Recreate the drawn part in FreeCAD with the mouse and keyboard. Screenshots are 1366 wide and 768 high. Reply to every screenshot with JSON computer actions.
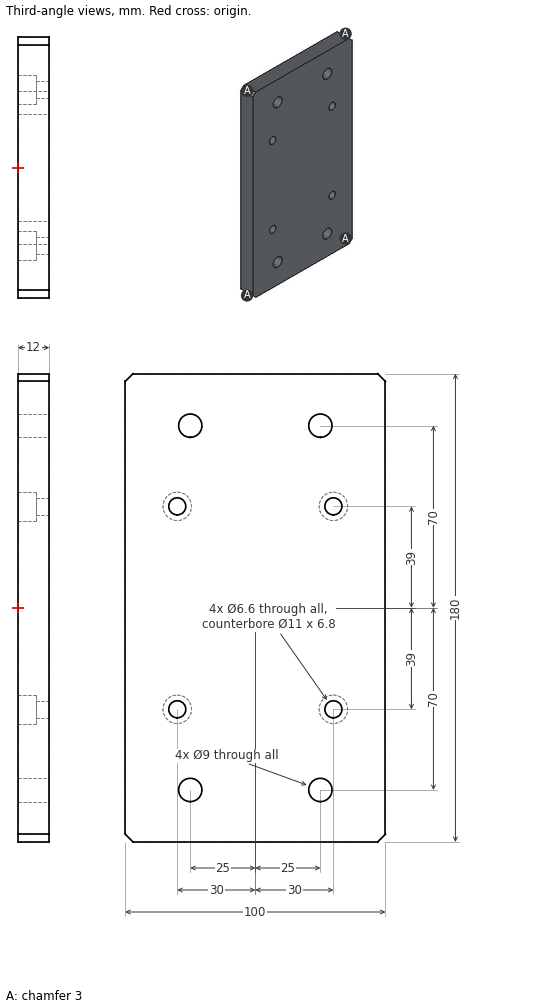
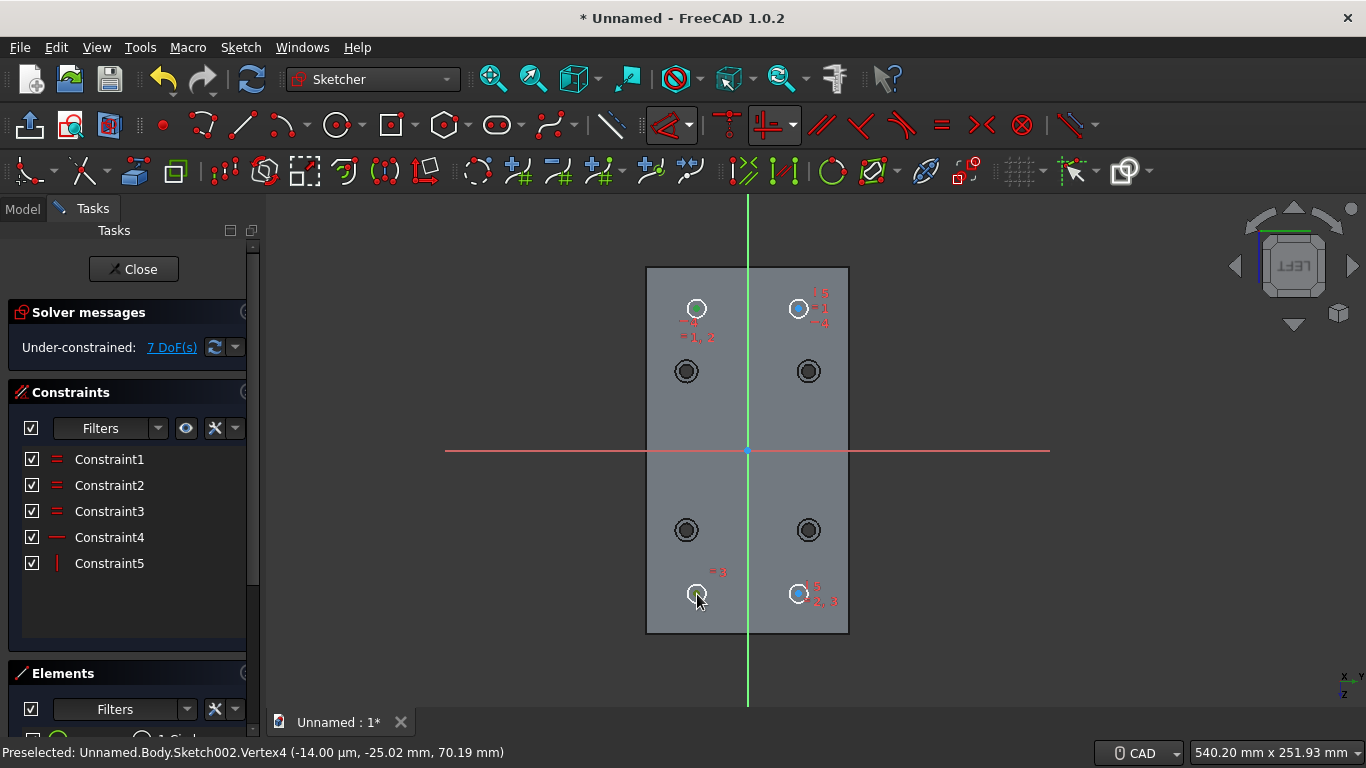
{"action": "left_click", "coordinate": [796, 126]}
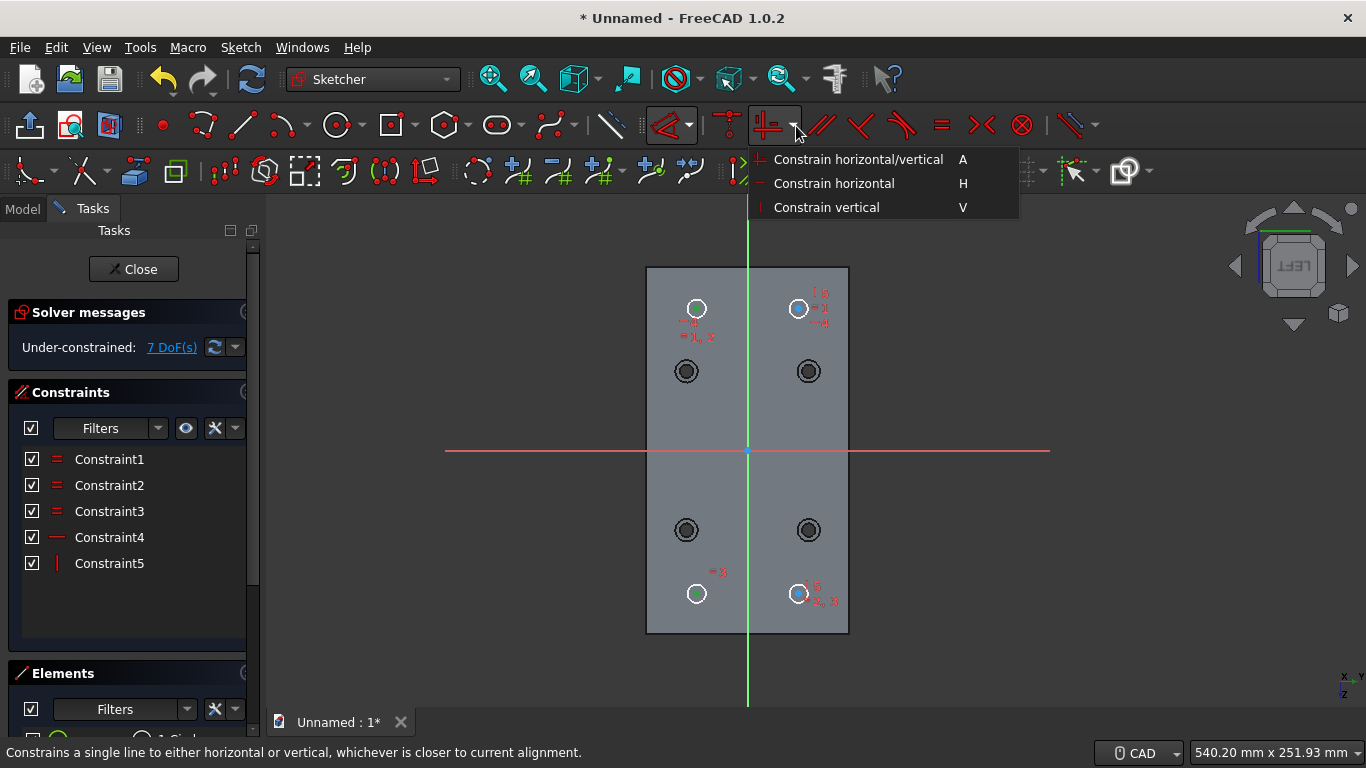
{"action": "left_click", "coordinate": [884, 207]}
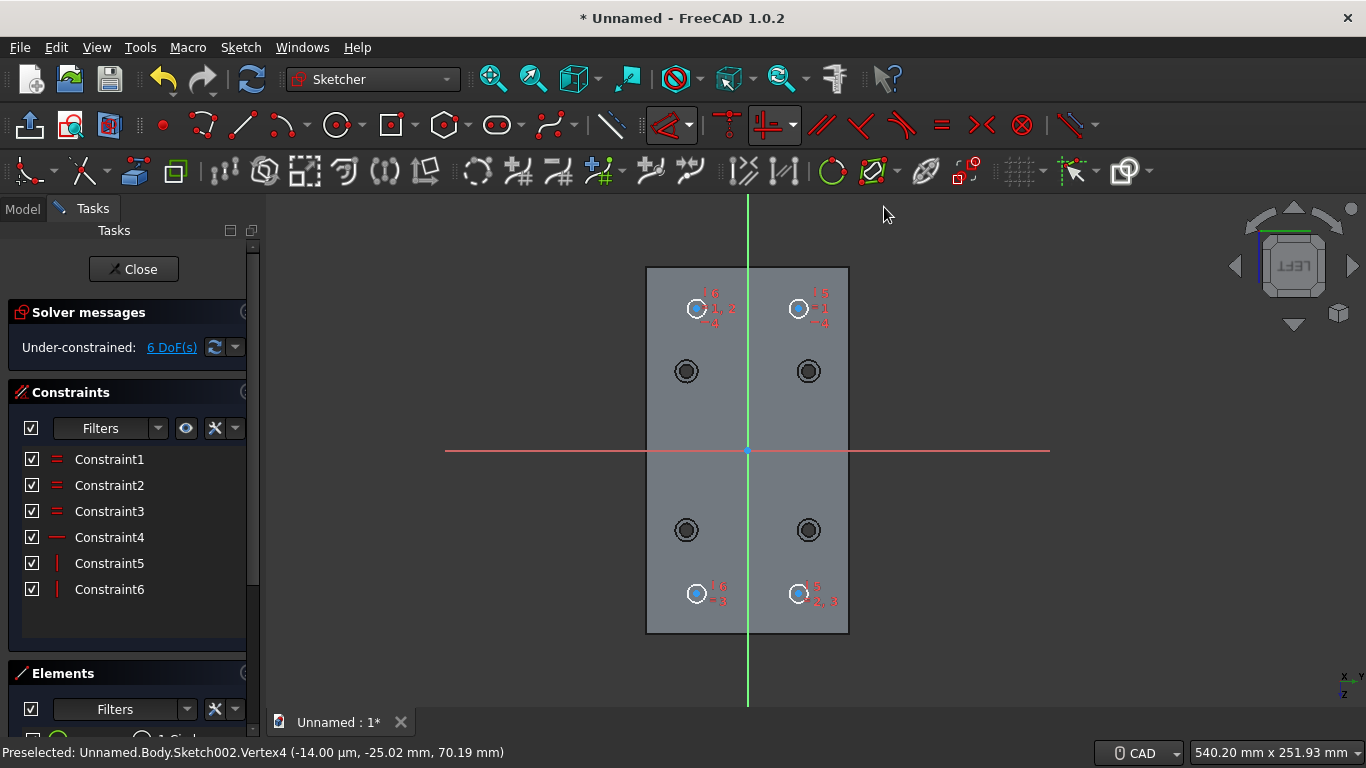
{"action": "left_click", "coordinate": [799, 594]}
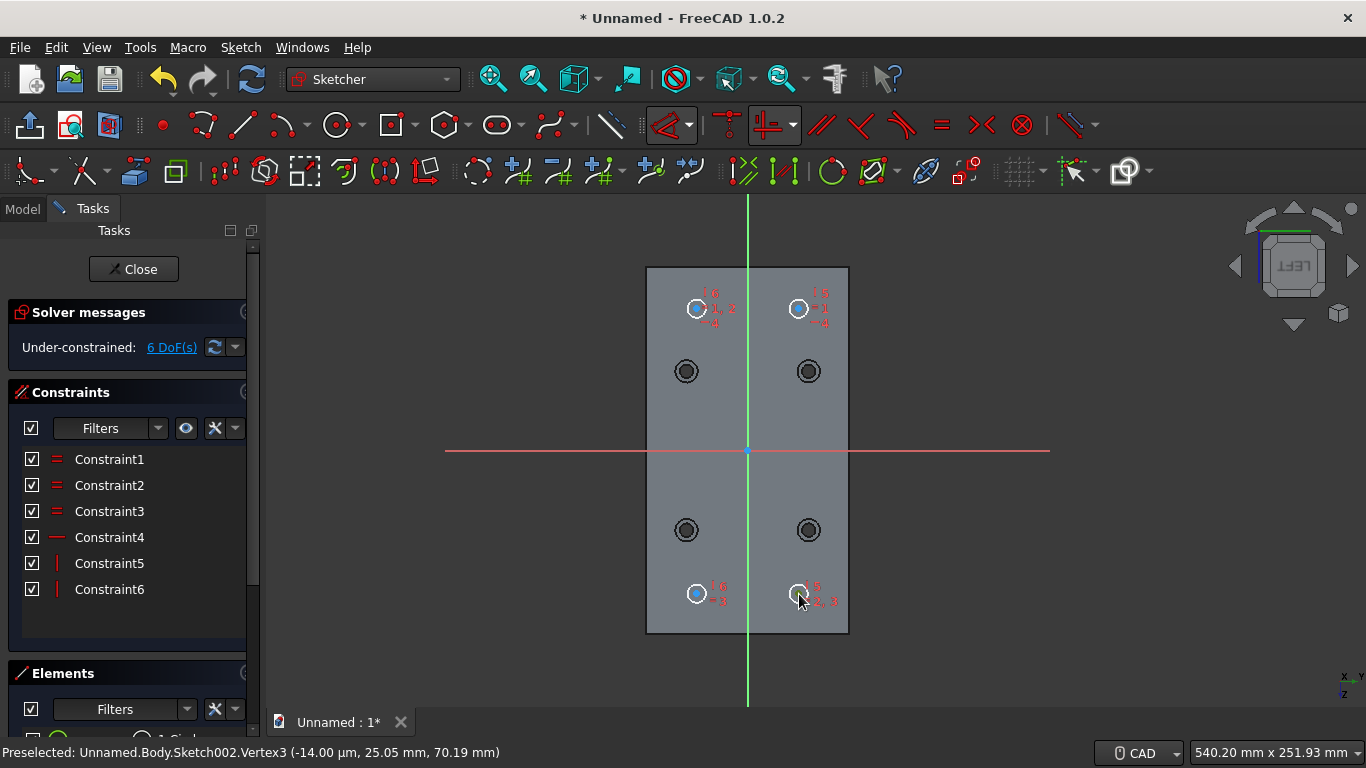
{"action": "left_click", "coordinate": [697, 594]}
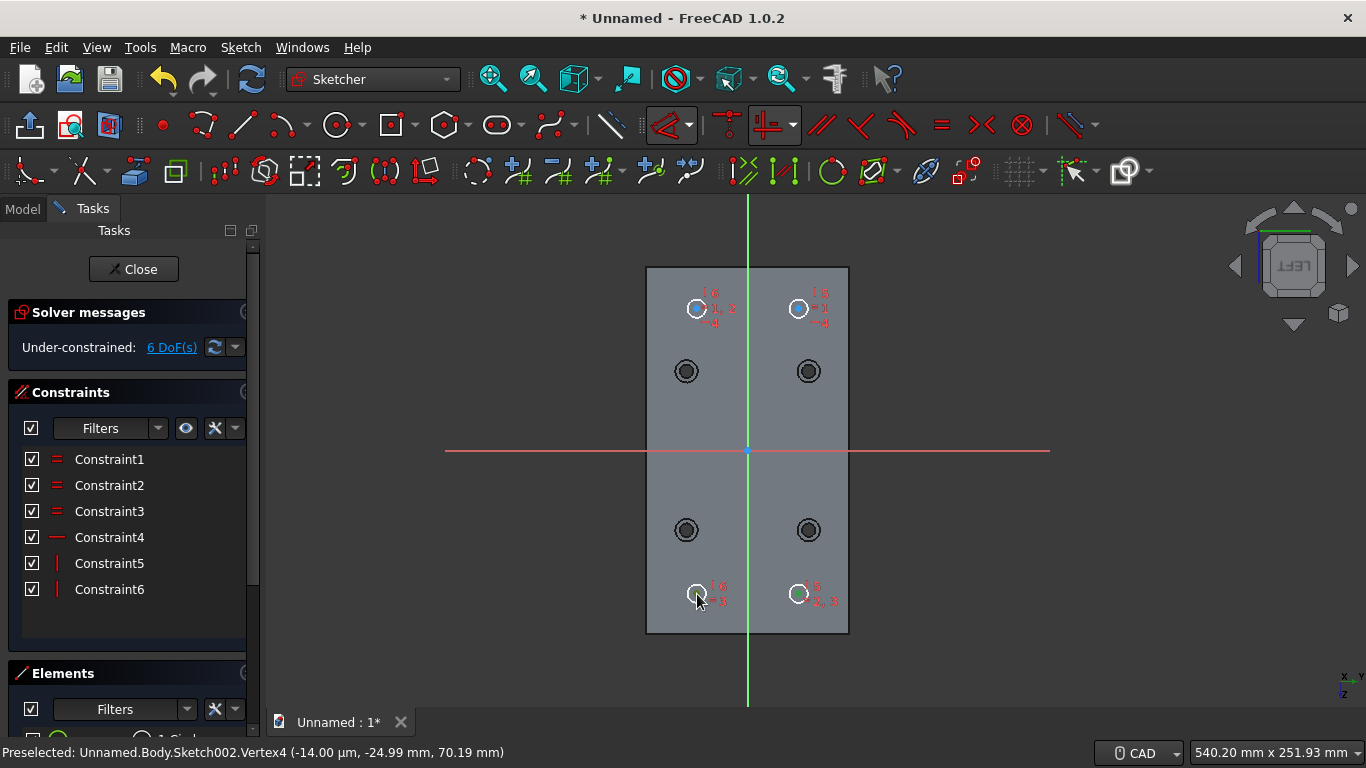
{"action": "key", "text": "h"}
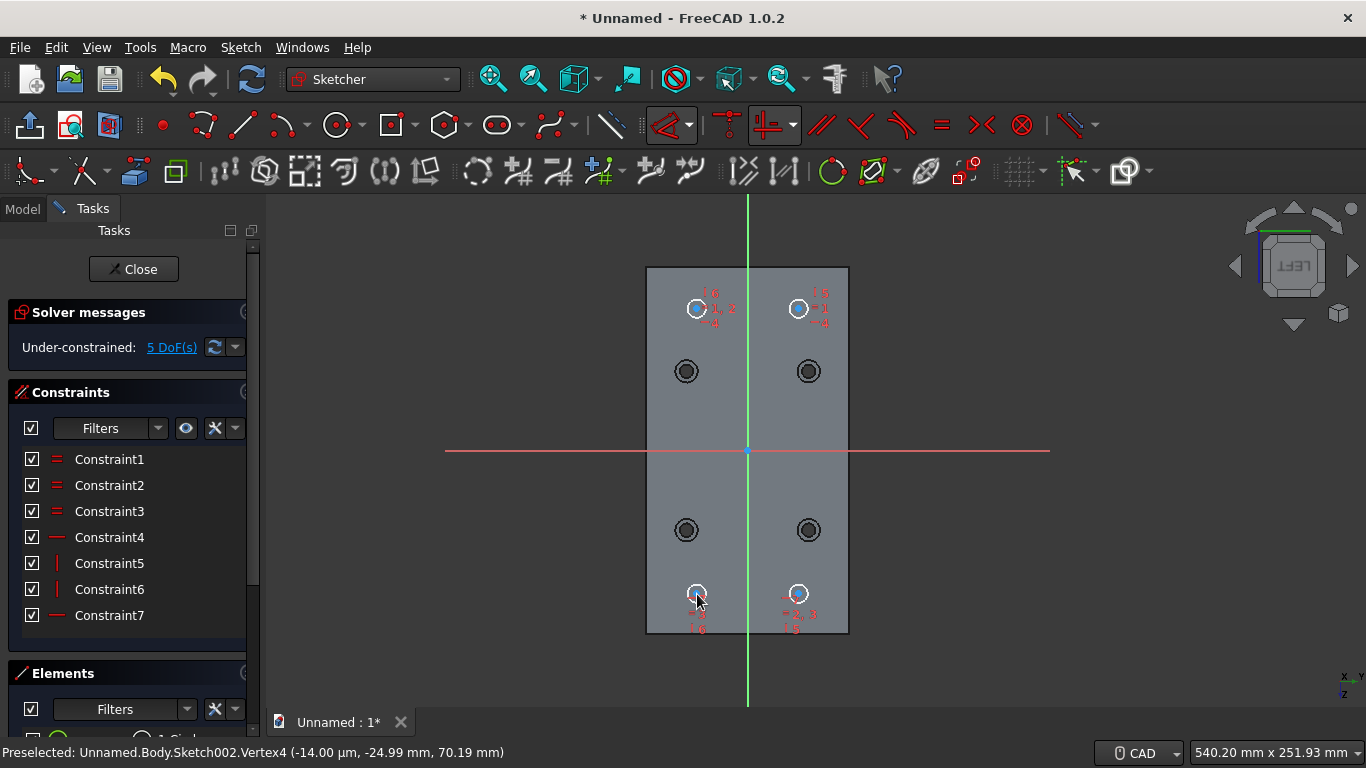
{"action": "scroll", "coordinate": [805, 302], "scroll_direction": "up", "scroll_amount": 4}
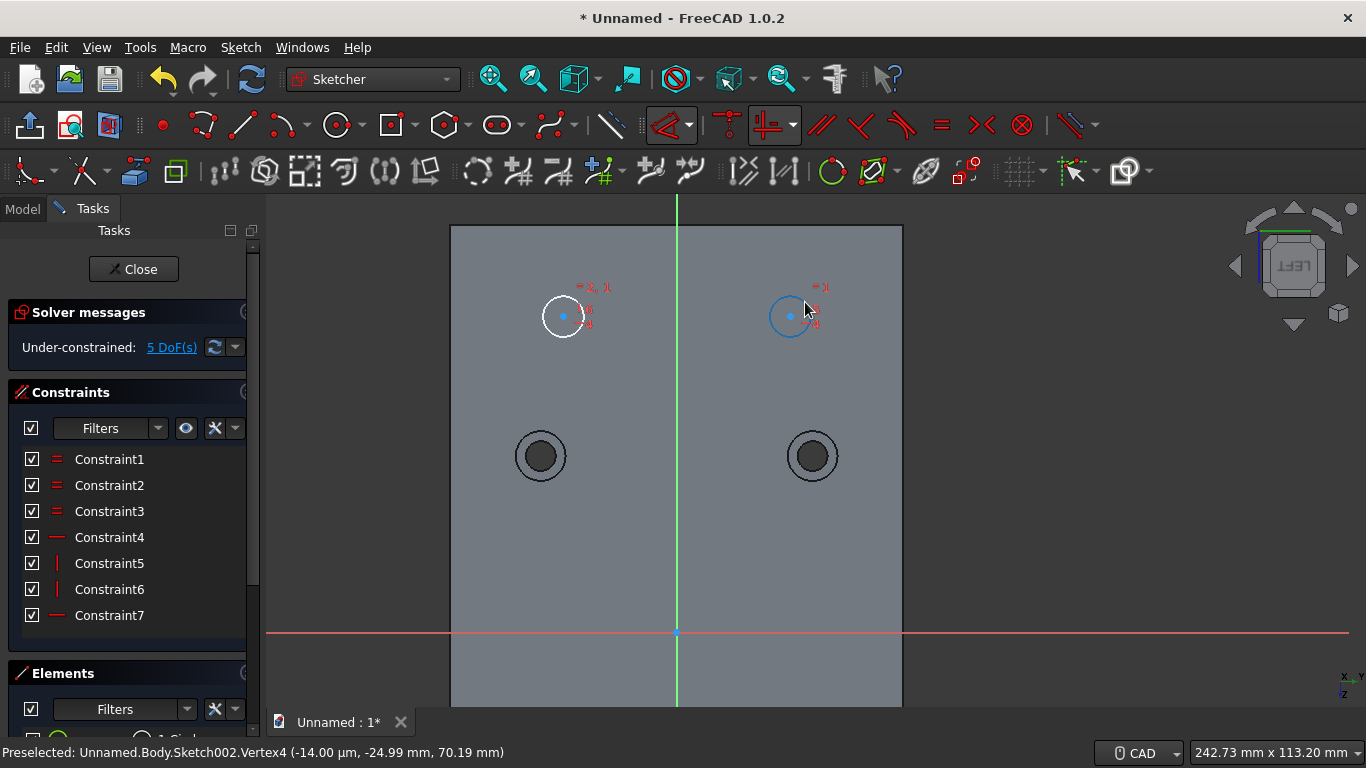
{"action": "left_click", "coordinate": [776, 302]}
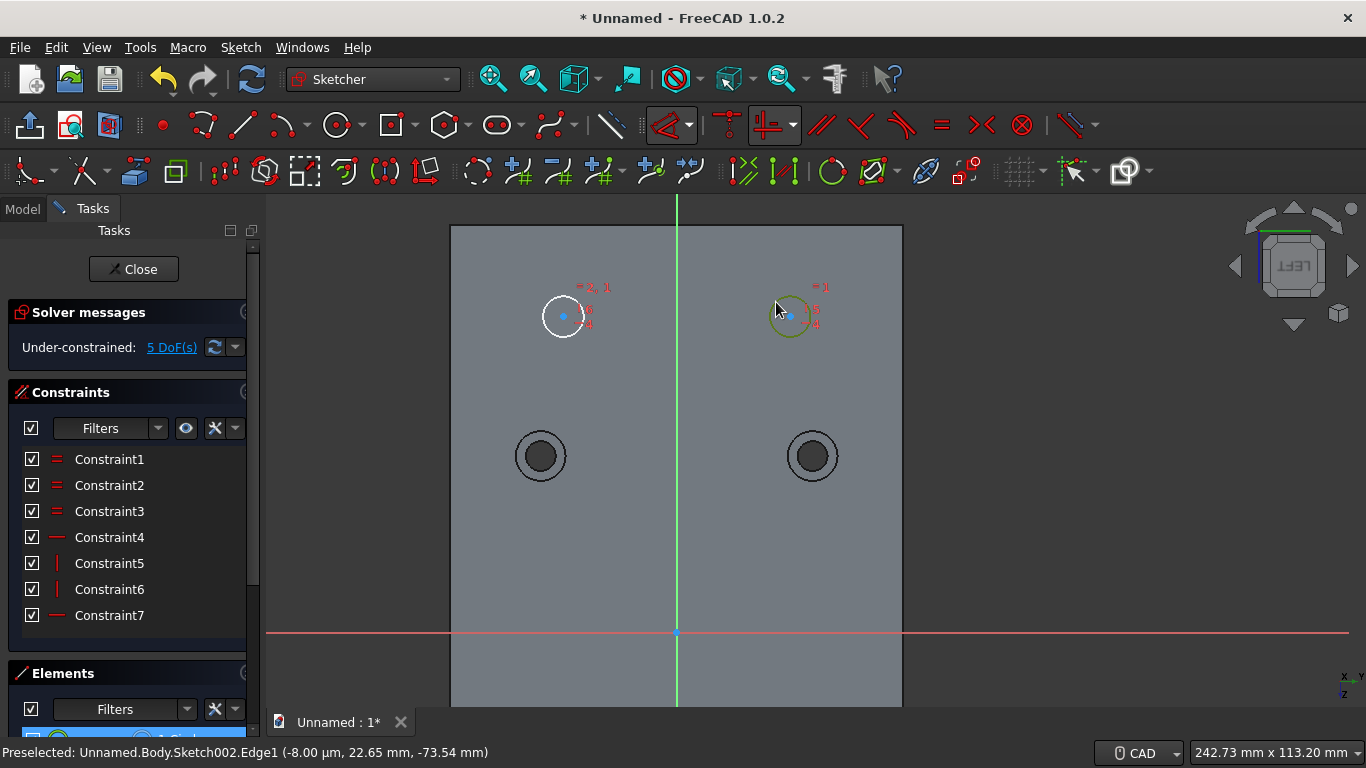
{"action": "key", "text": "k o"}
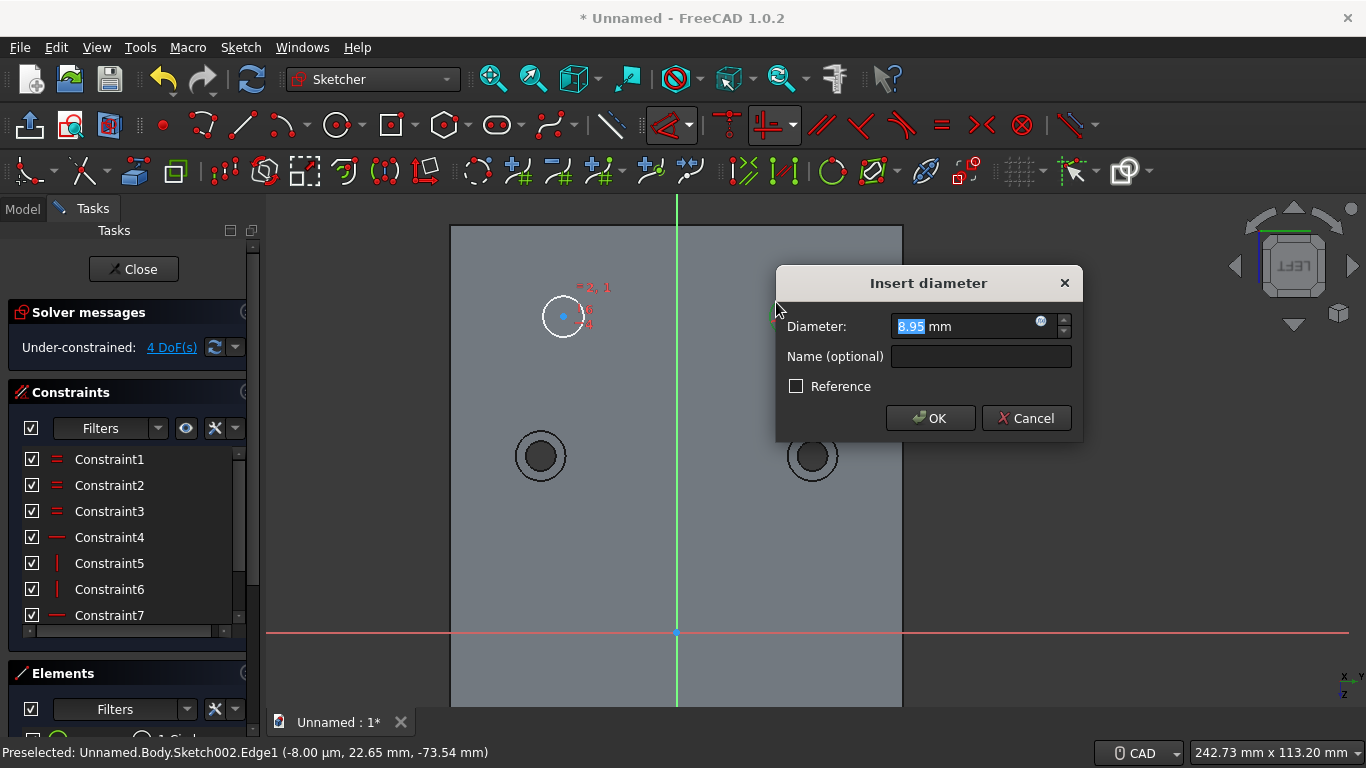
{"action": "type", "text": "9"}
{"action": "key", "text": "Return"}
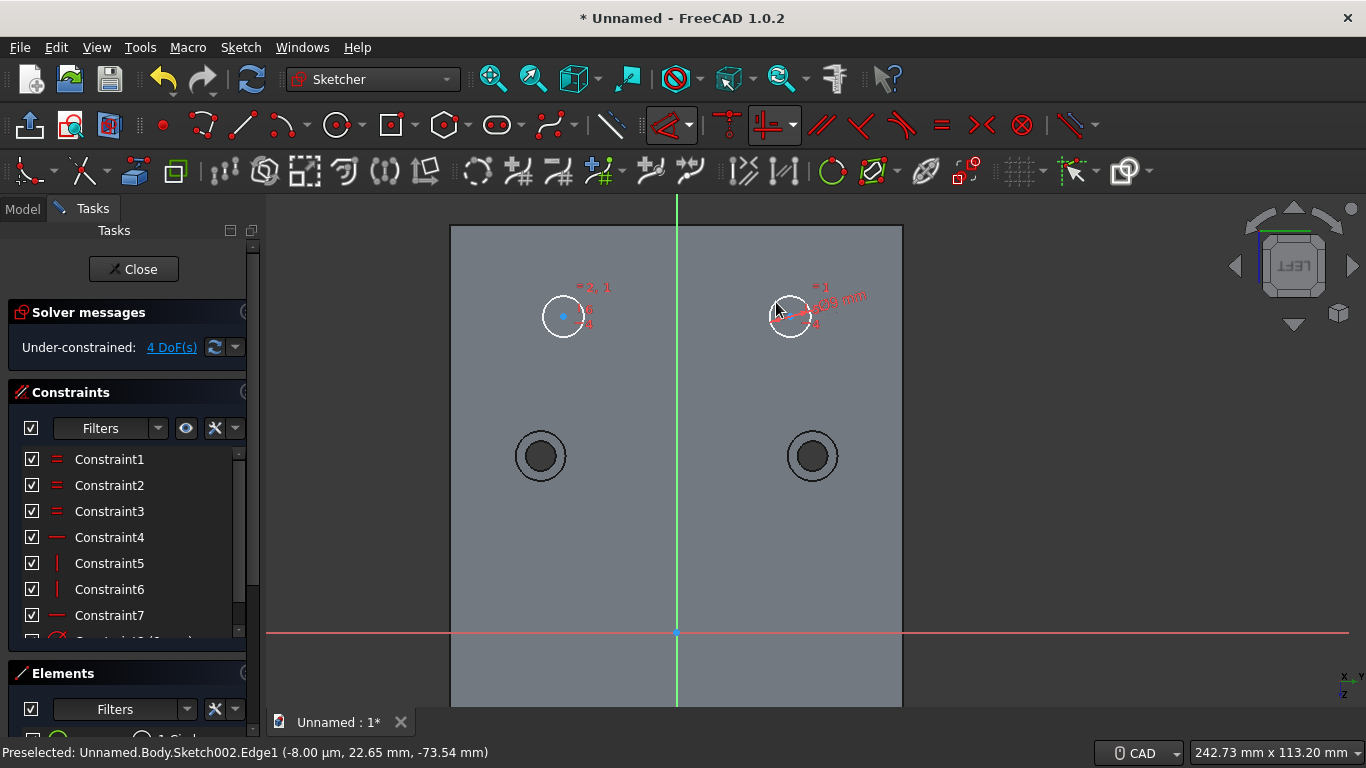
{"action": "left_click", "coordinate": [790, 317]}